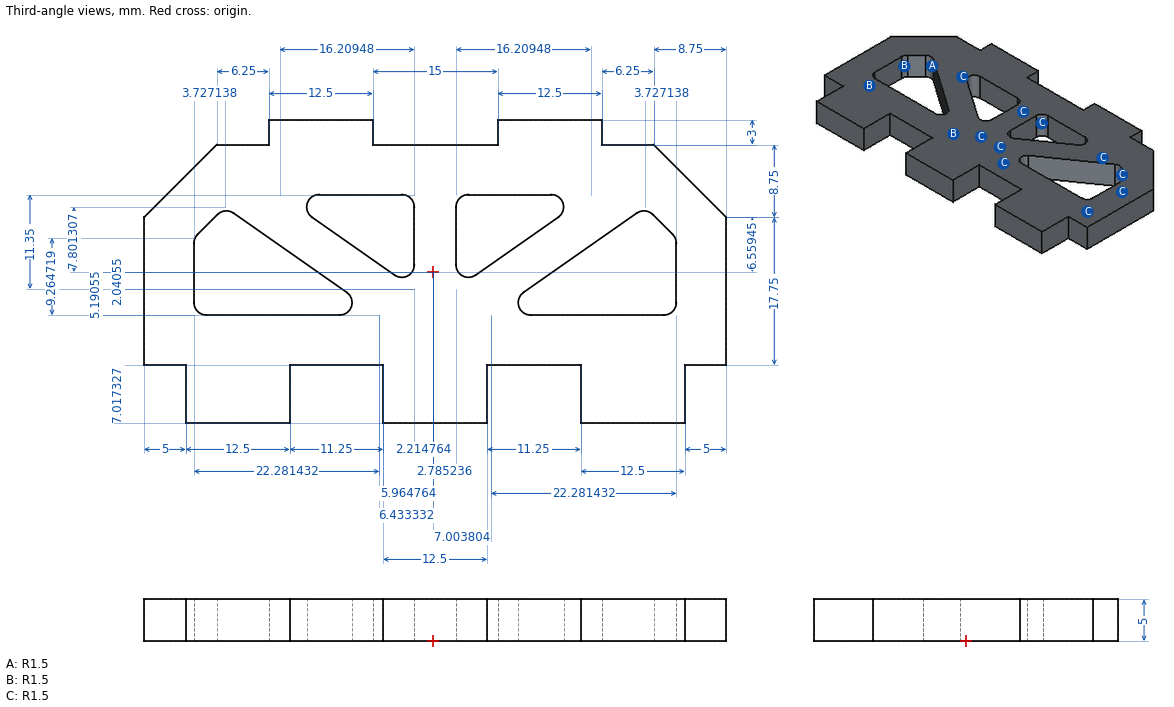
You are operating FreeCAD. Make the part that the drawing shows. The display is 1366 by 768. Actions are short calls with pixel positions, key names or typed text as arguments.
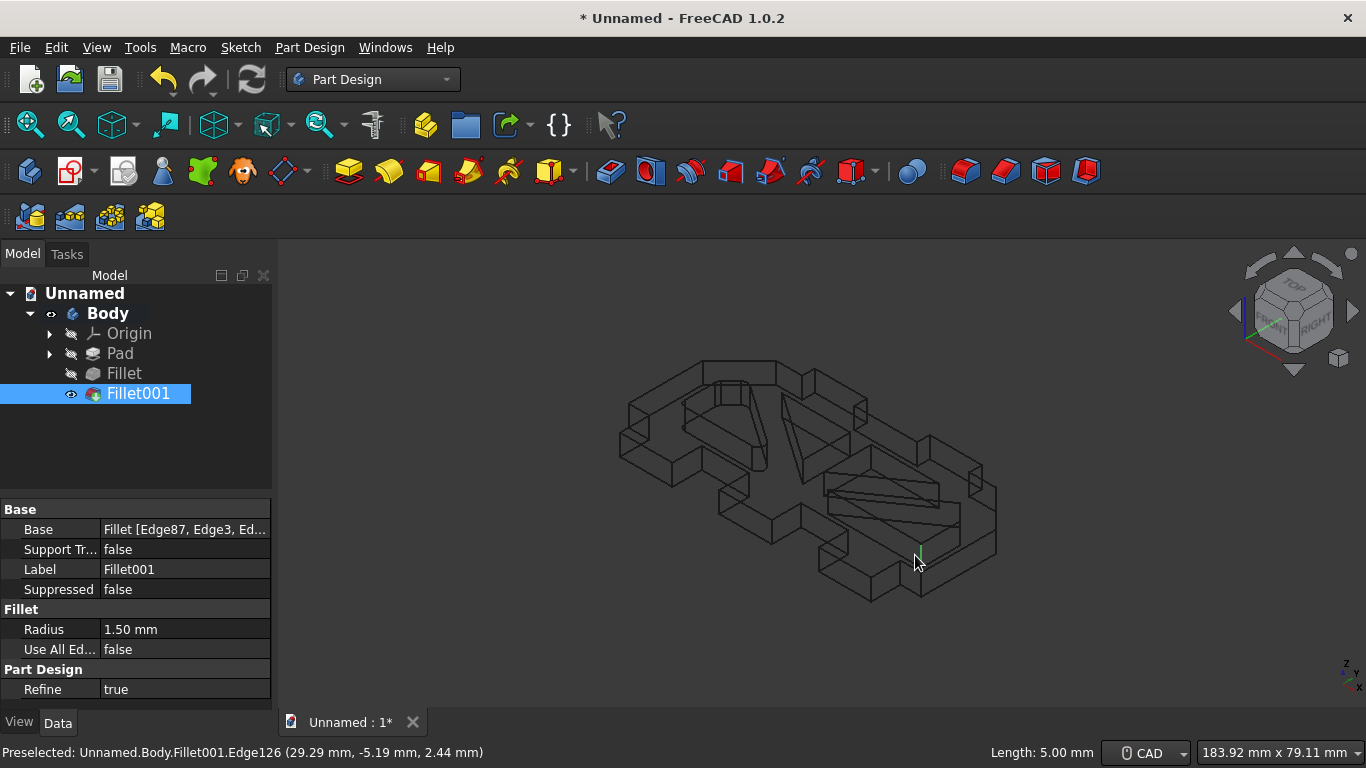
click(960, 532, ctrl)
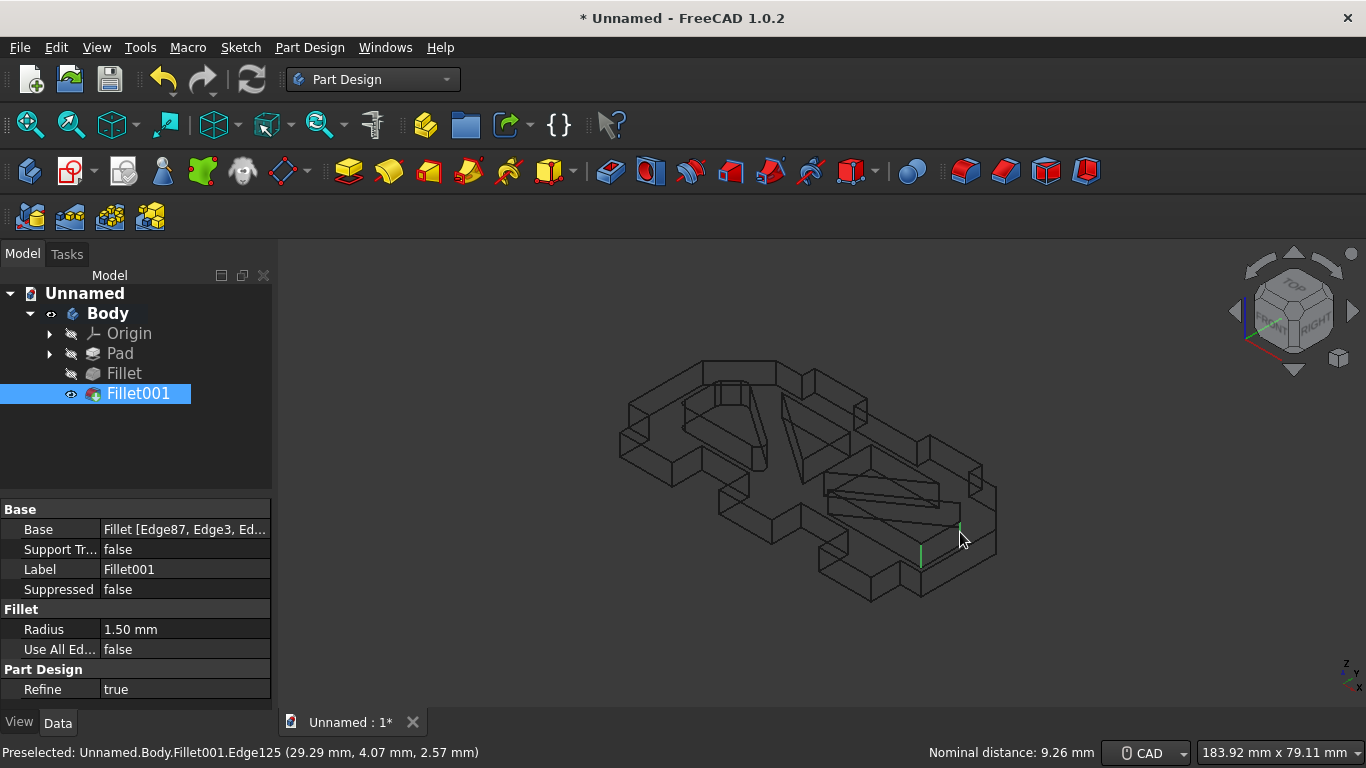
click(782, 414, ctrl)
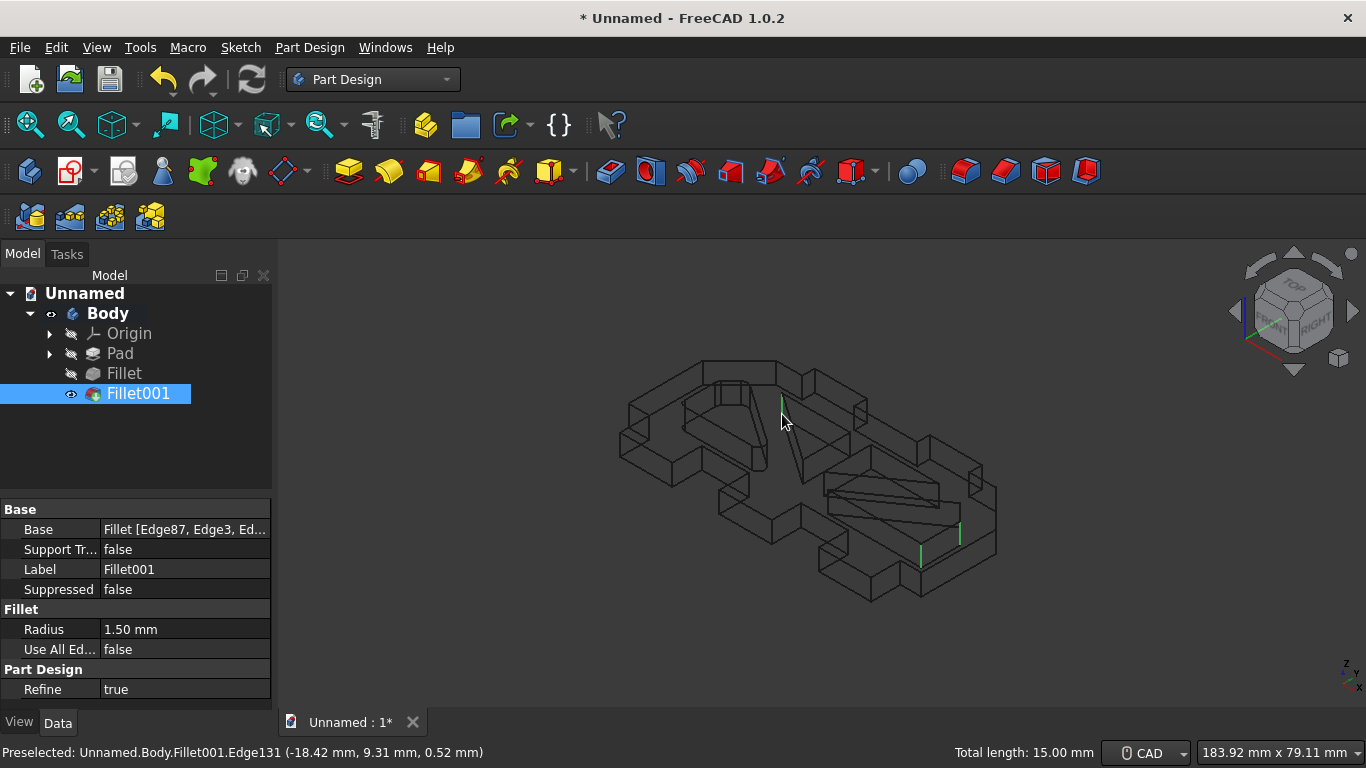
click(803, 471, ctrl)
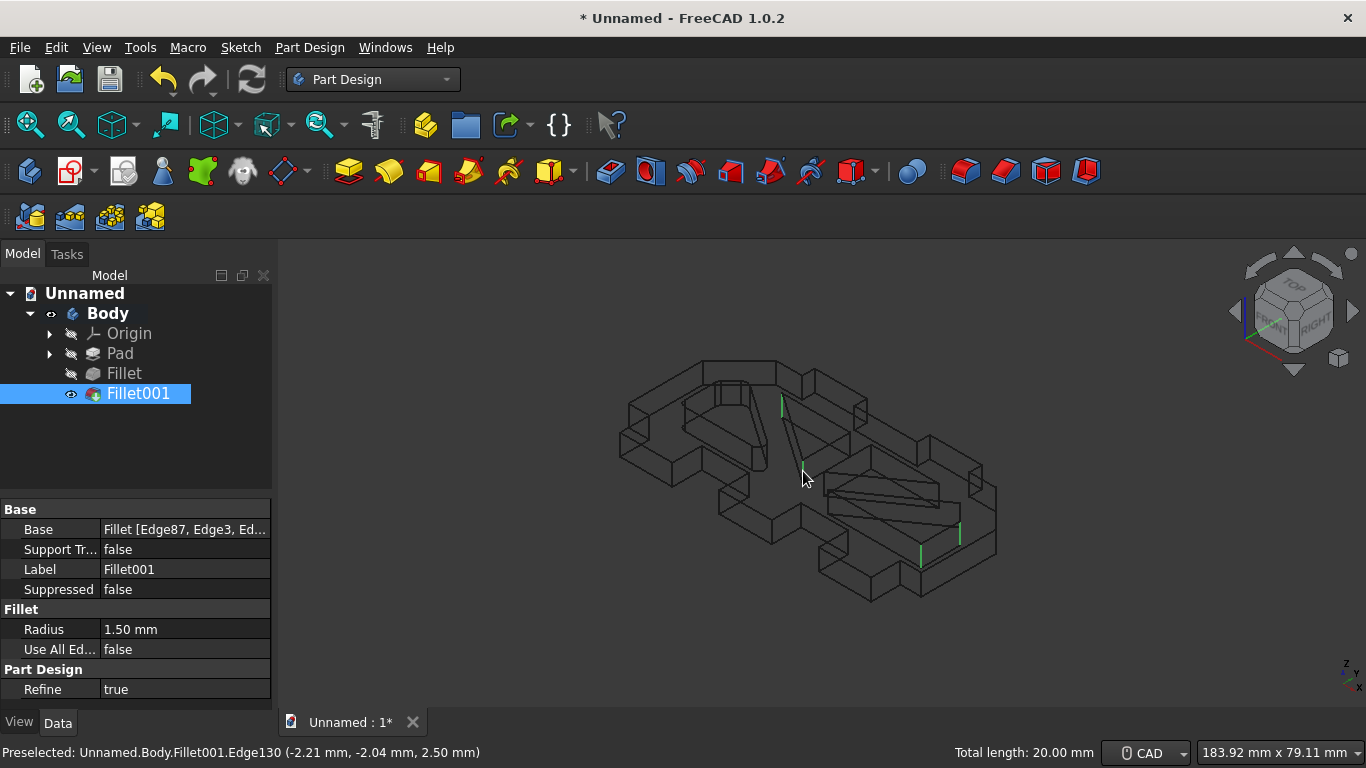
click(850, 444, ctrl)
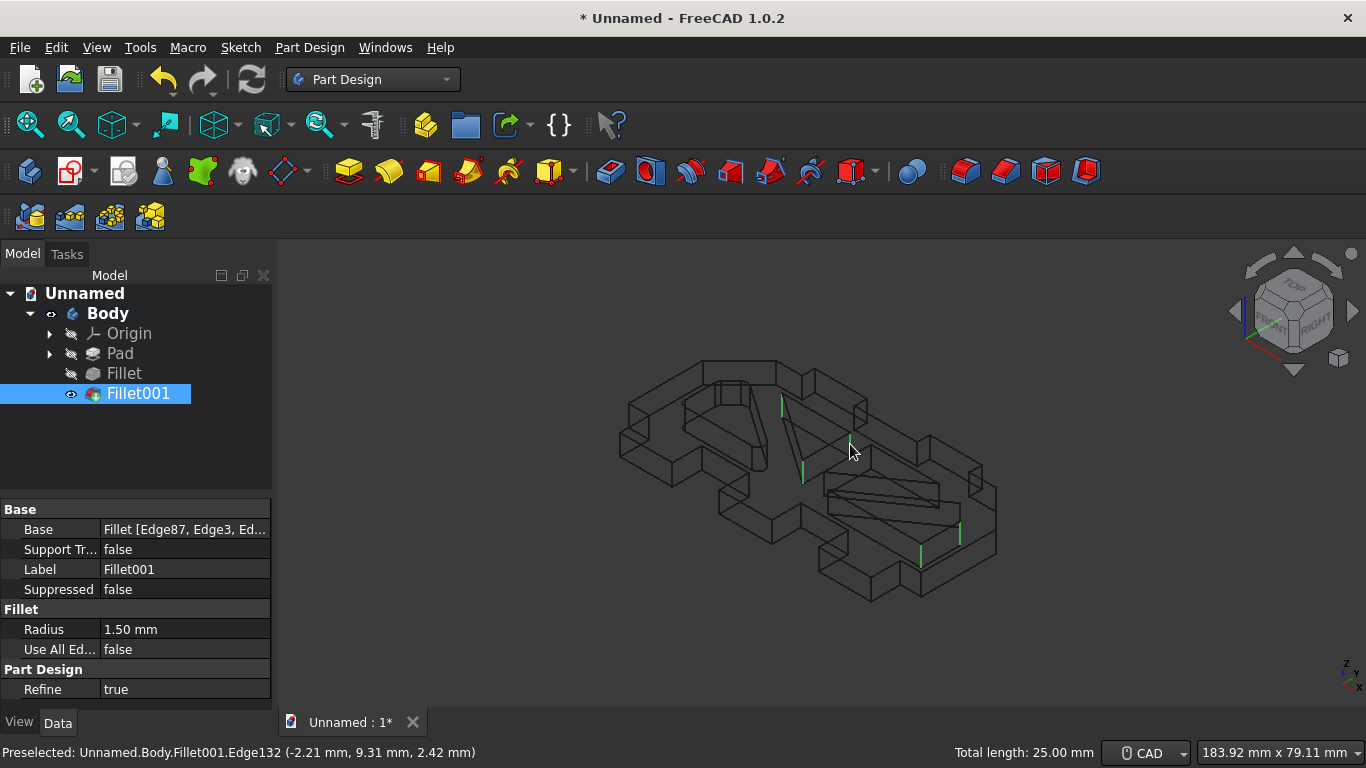
click(871, 456, ctrl)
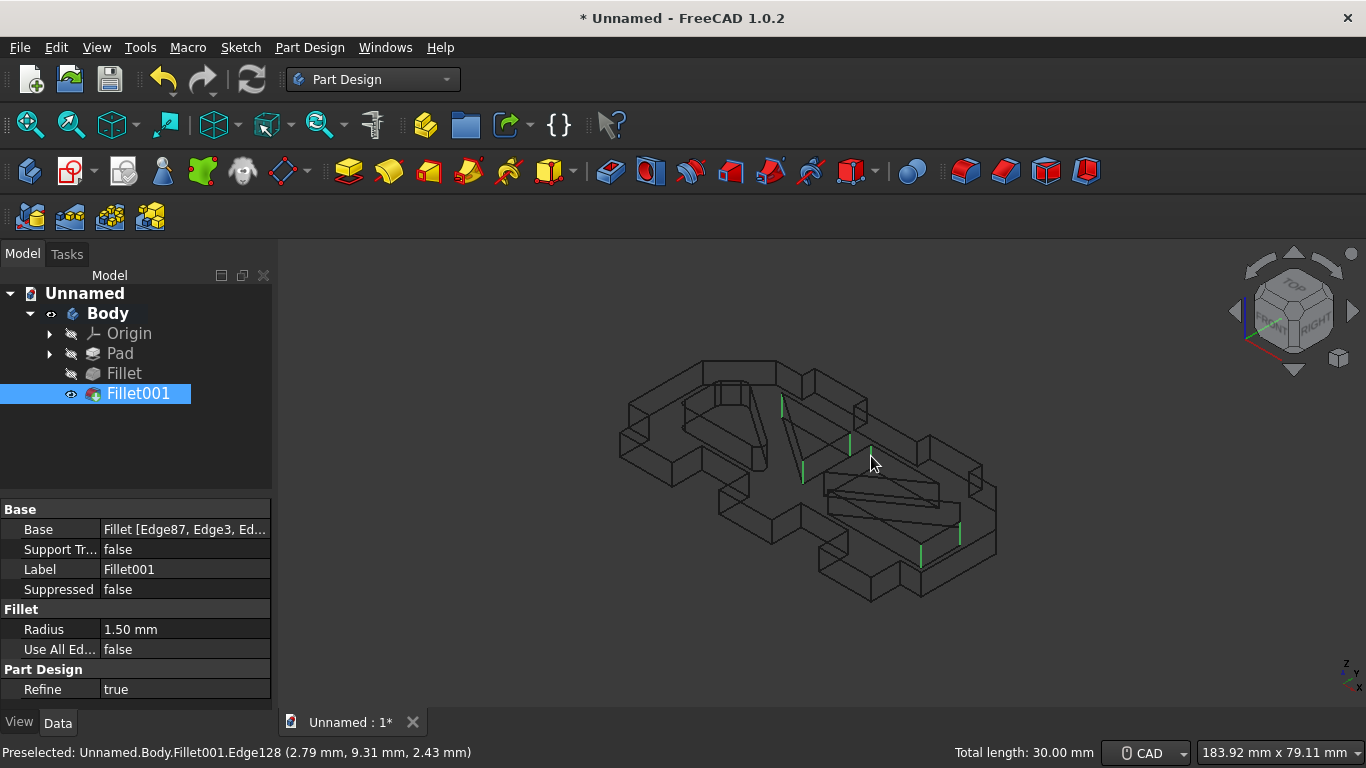
click(824, 483, ctrl)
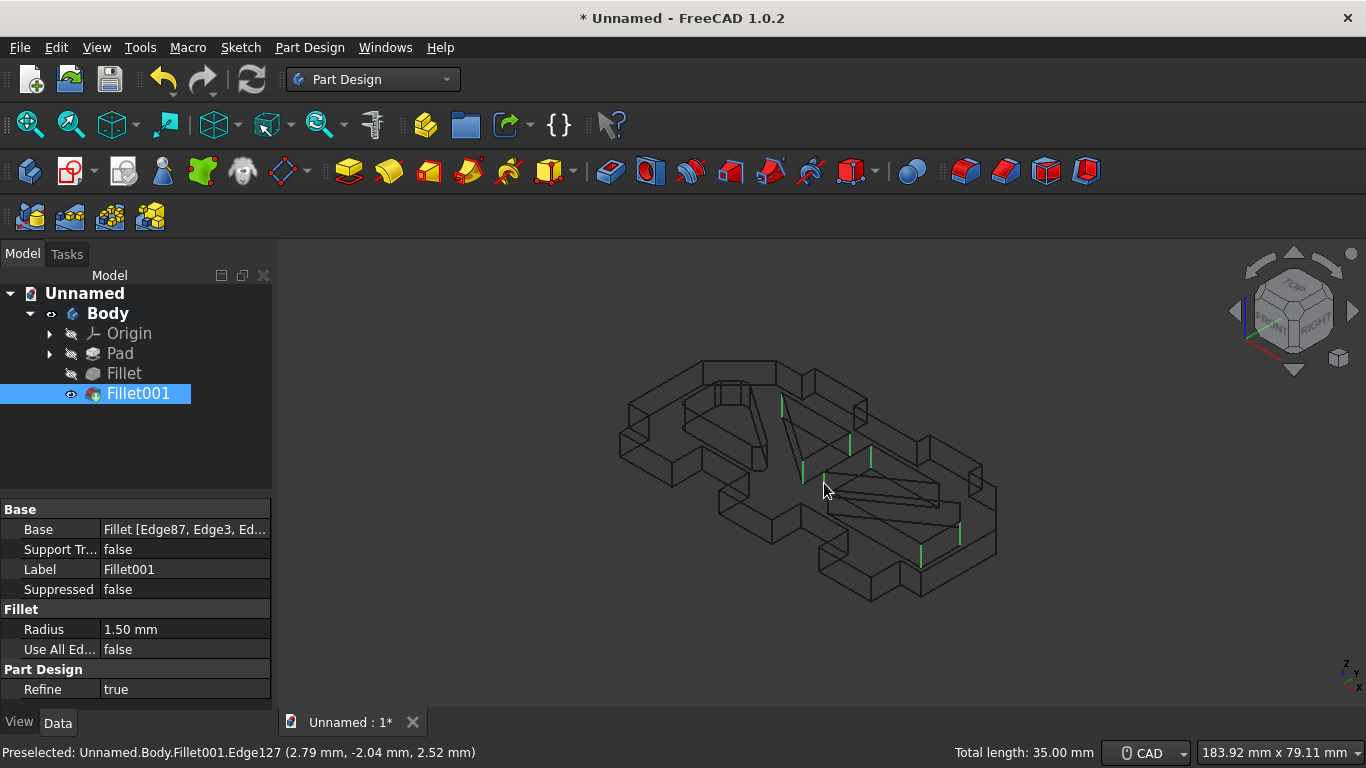
click(939, 492, ctrl)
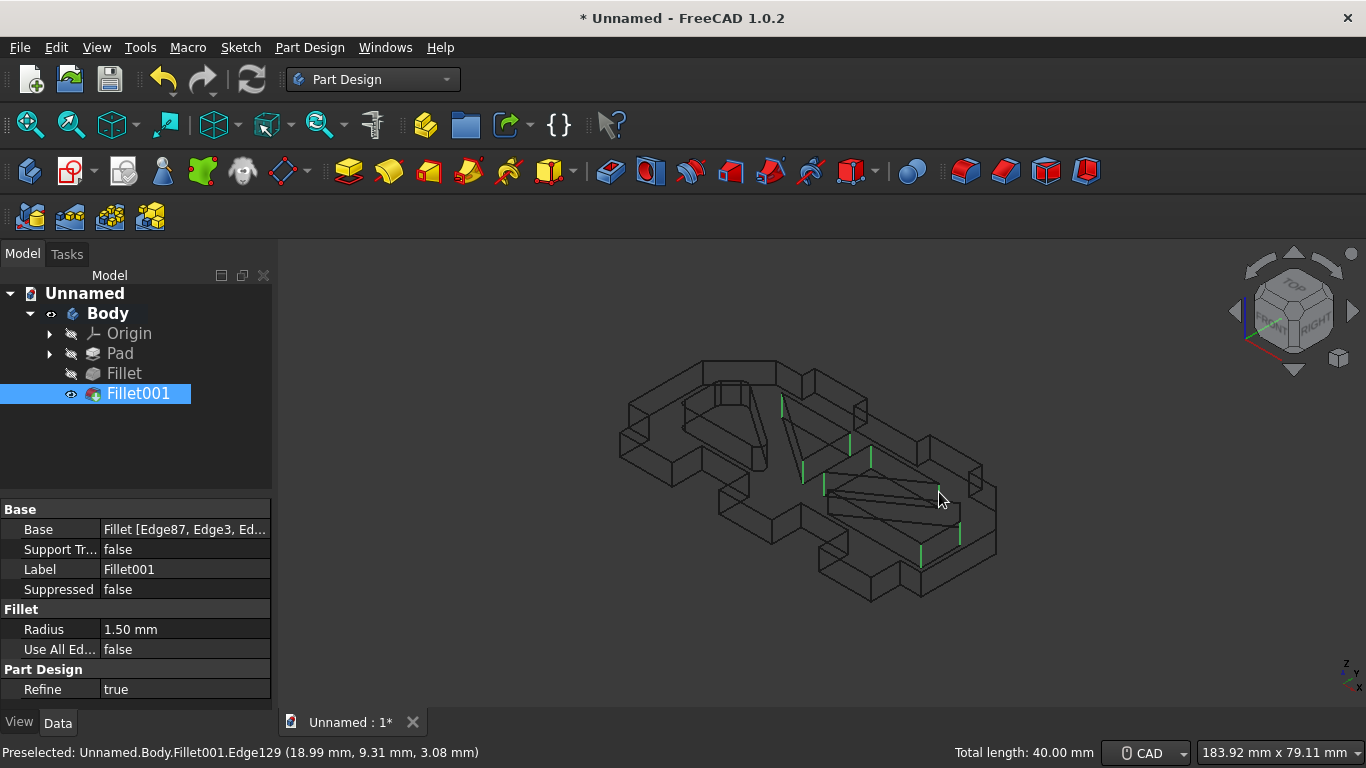
click(828, 501, ctrl)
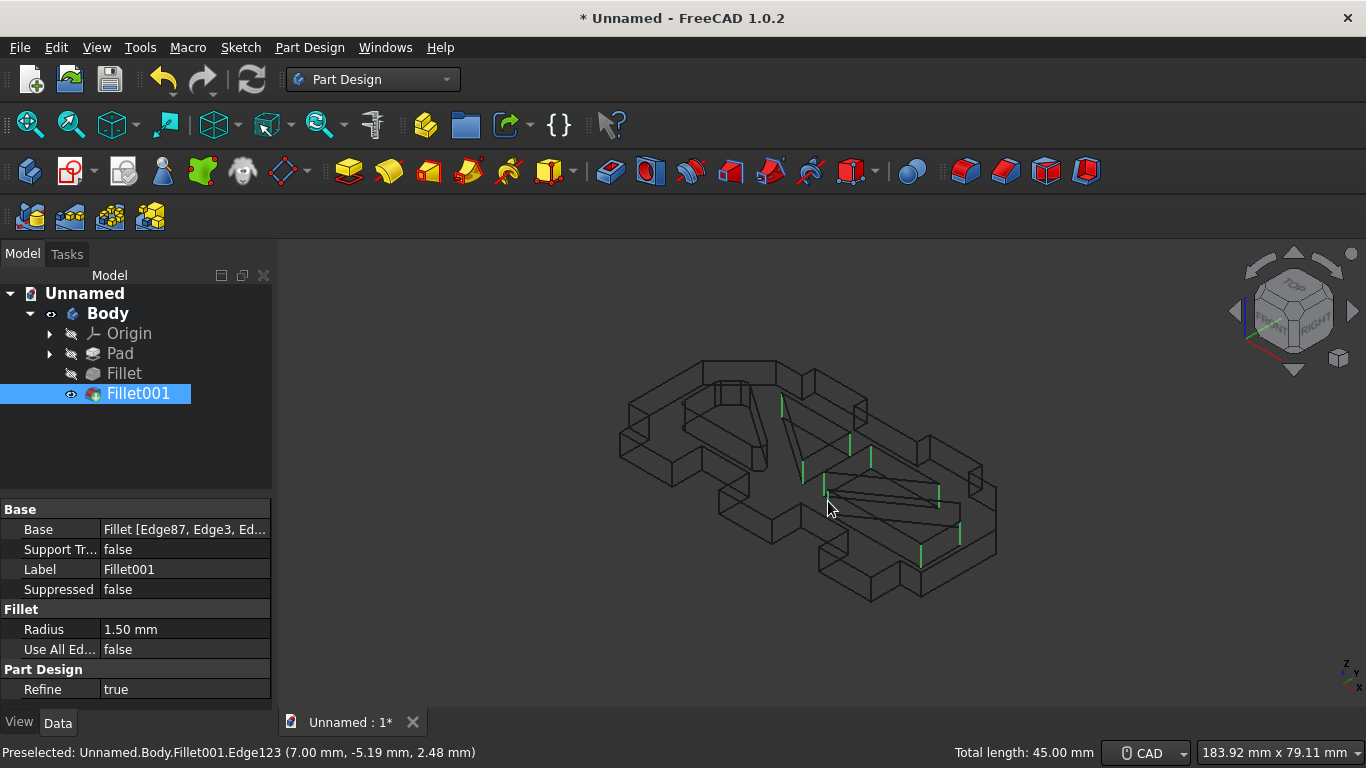
scroll(960, 514, up, 6)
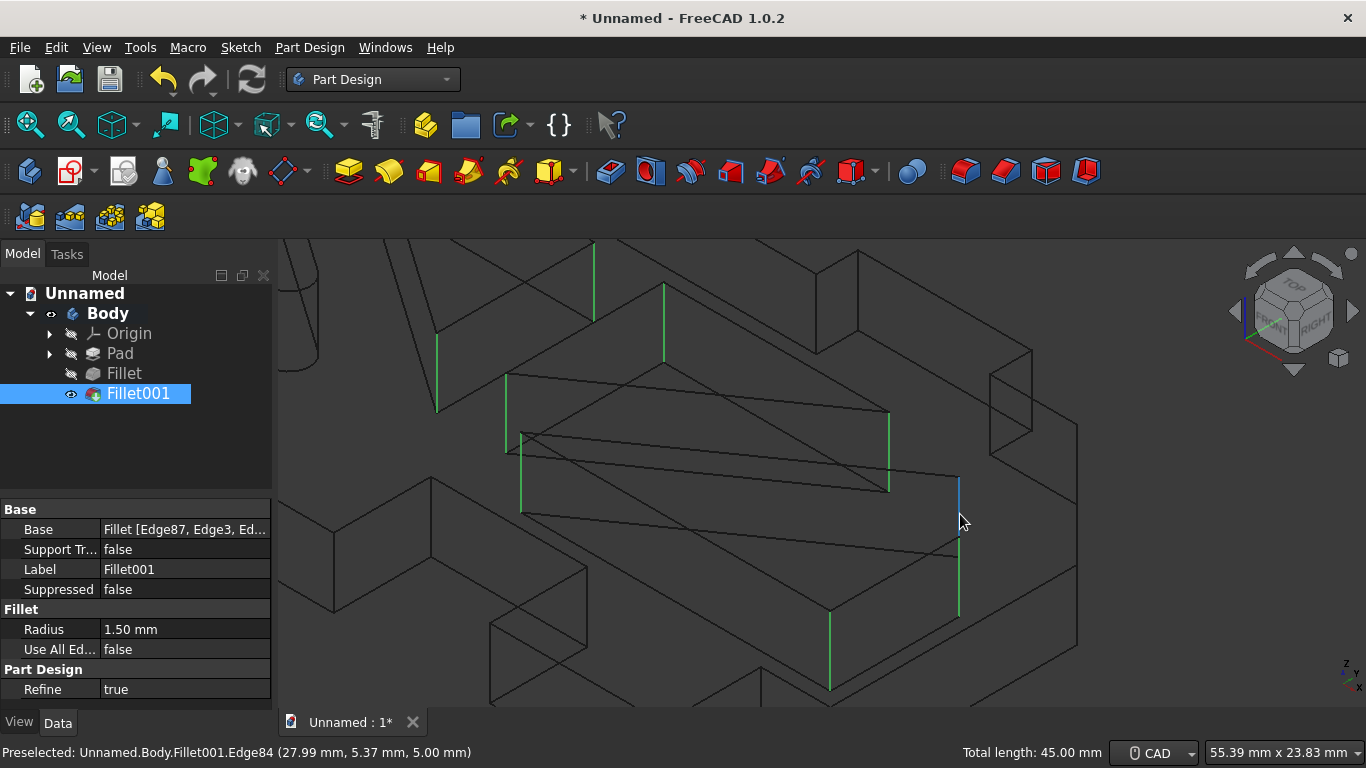
key(v)
key(f)